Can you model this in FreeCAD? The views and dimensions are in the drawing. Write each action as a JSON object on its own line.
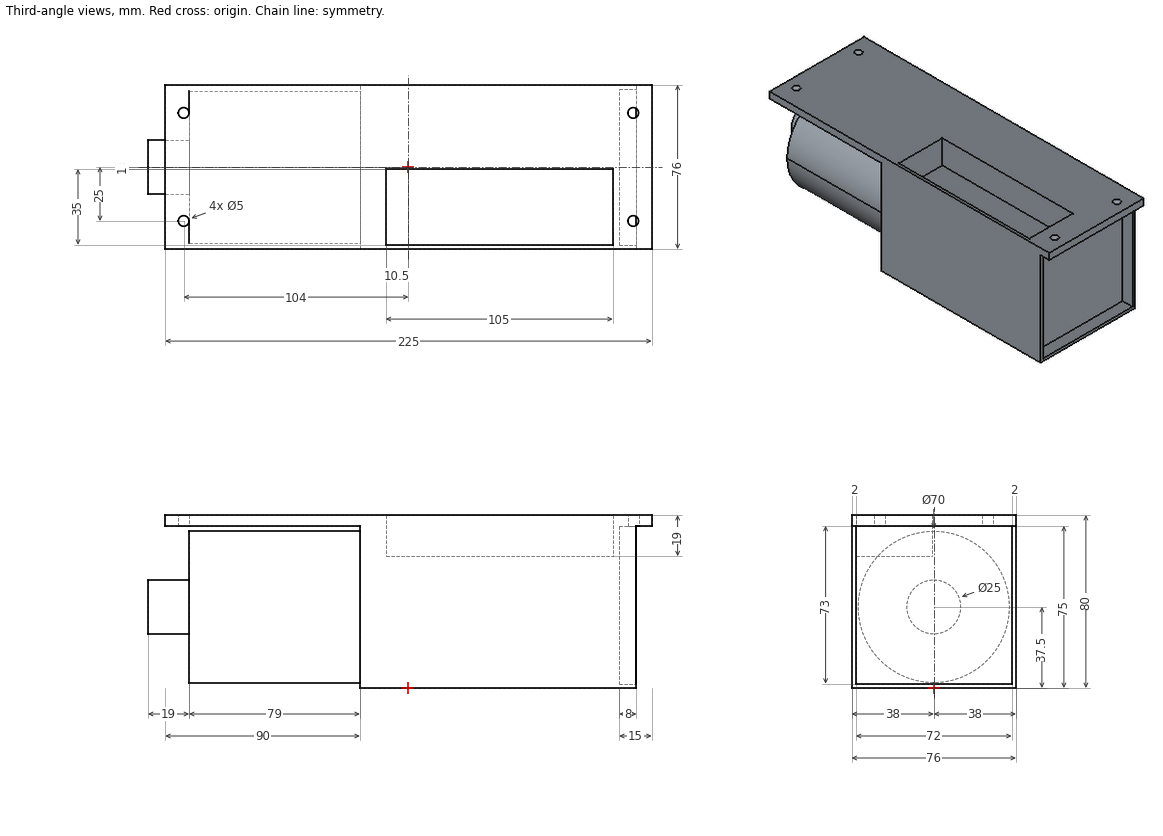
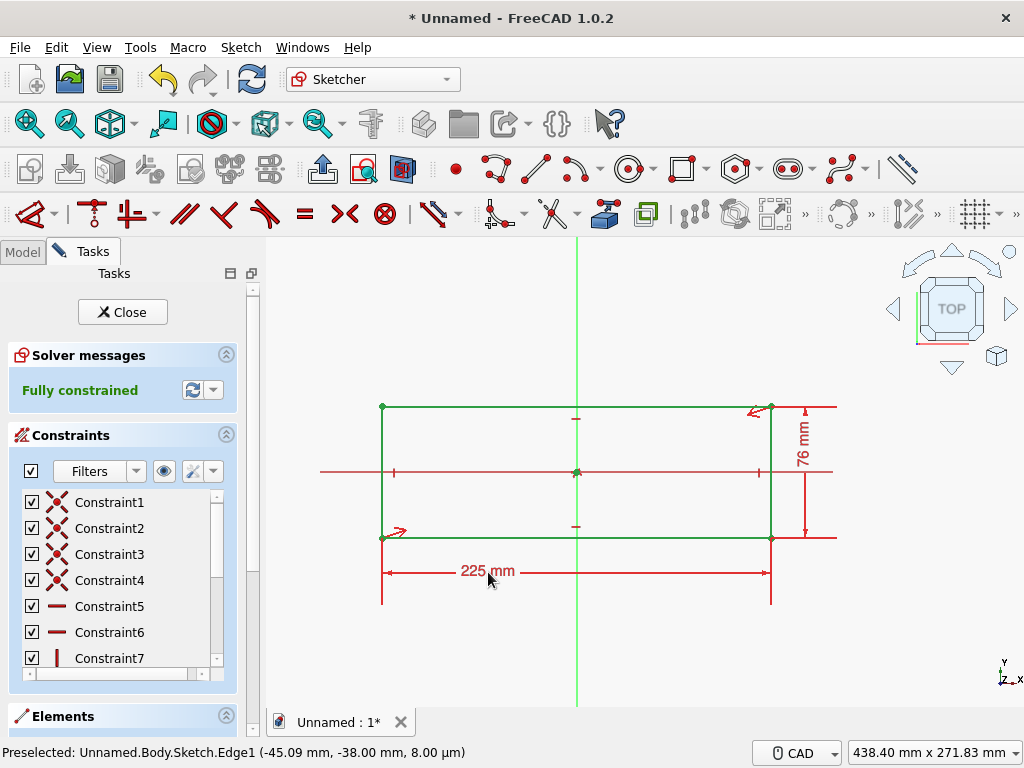
{"action": "left_click", "coordinate": [123, 312]}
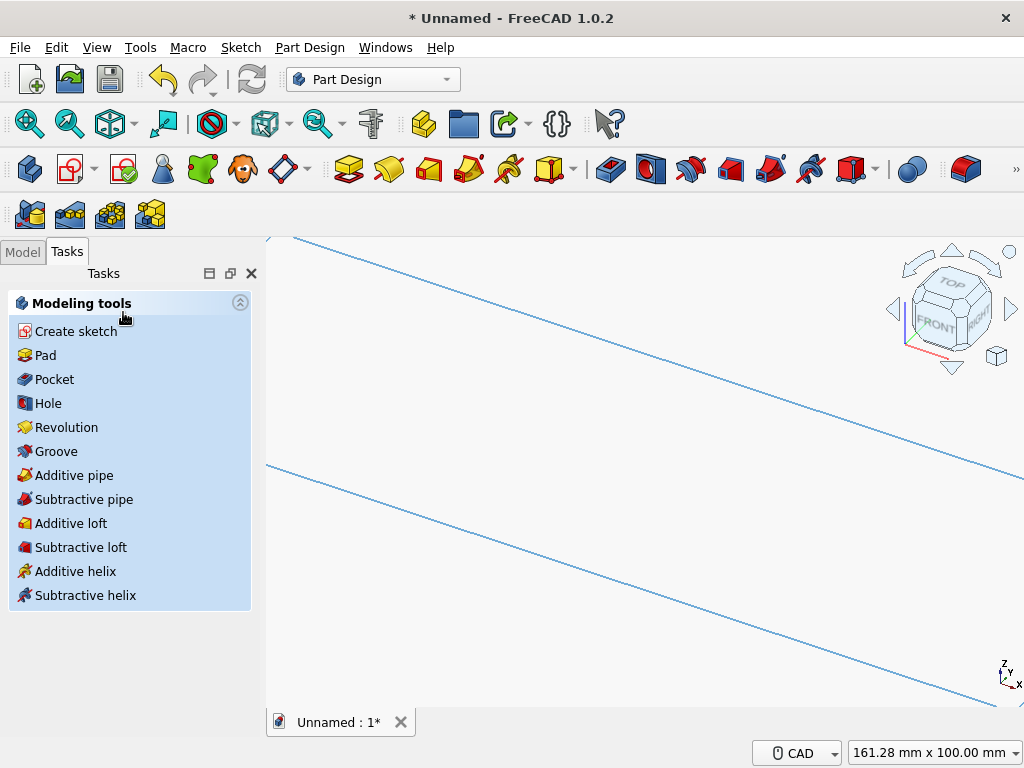
{"action": "left_click", "coordinate": [350, 170]}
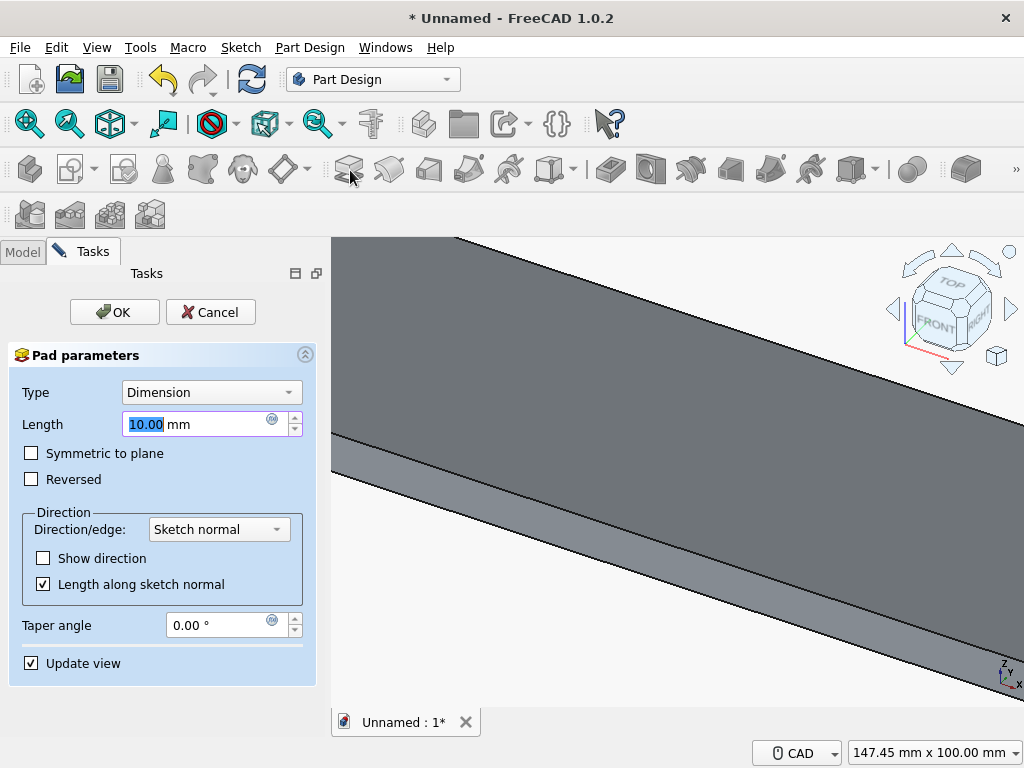
{"action": "type", "text": "80"}
{"action": "key", "text": "Tab"}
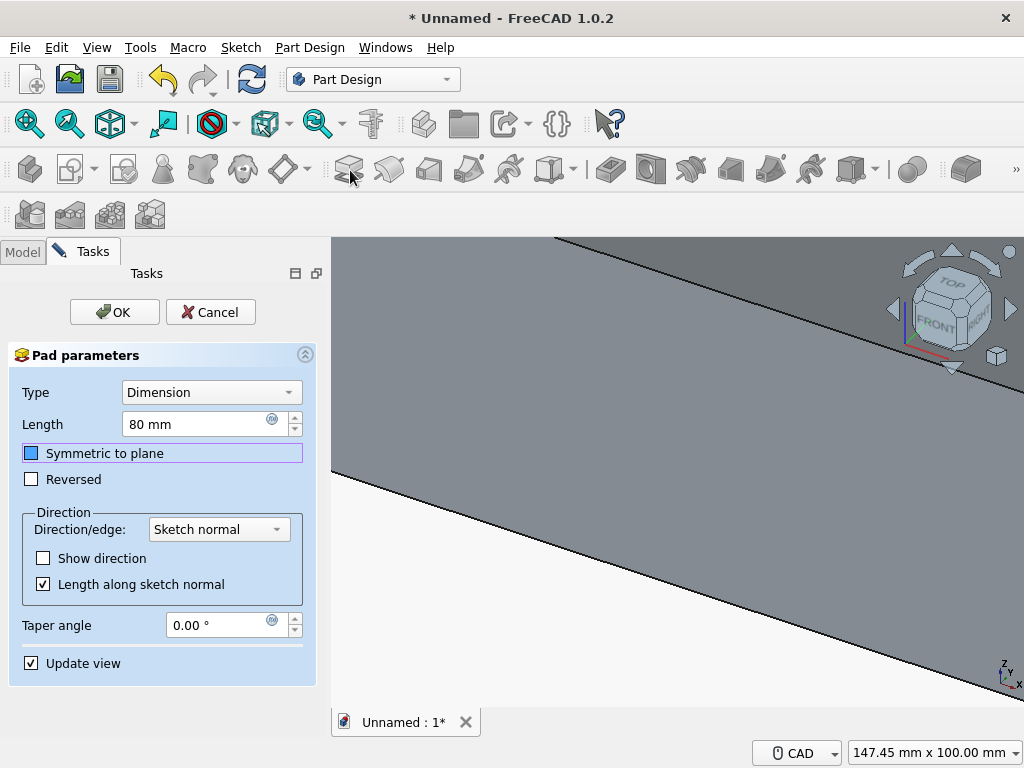
{"action": "left_click", "coordinate": [115, 312]}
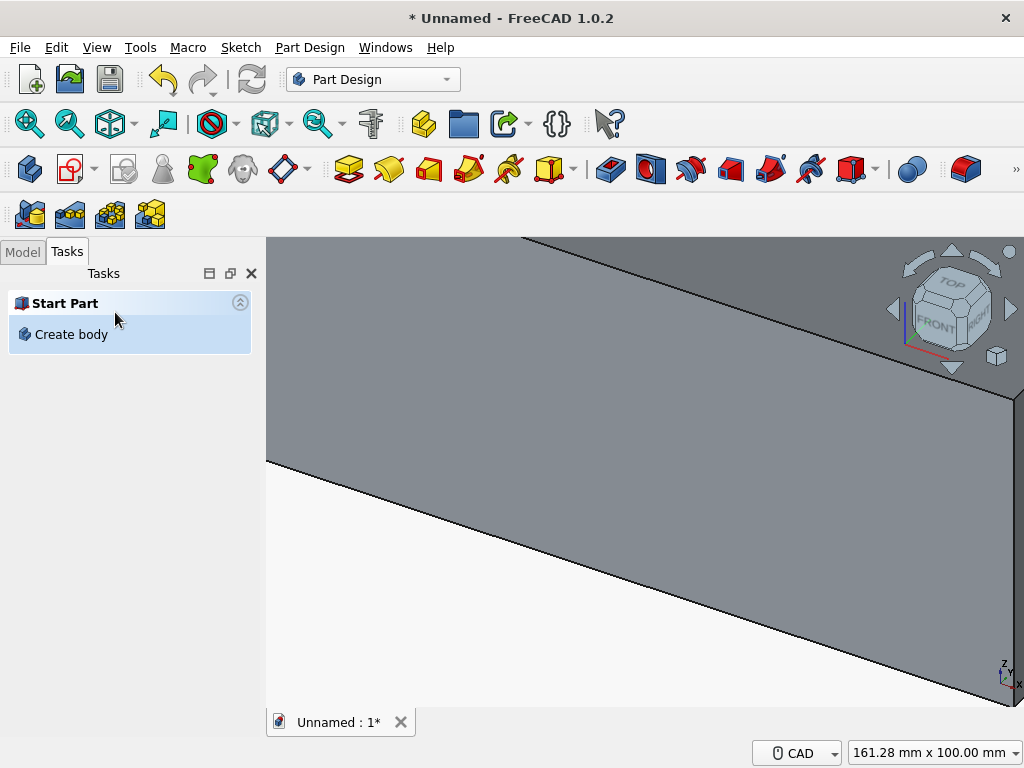
{"action": "key", "text": "v f"}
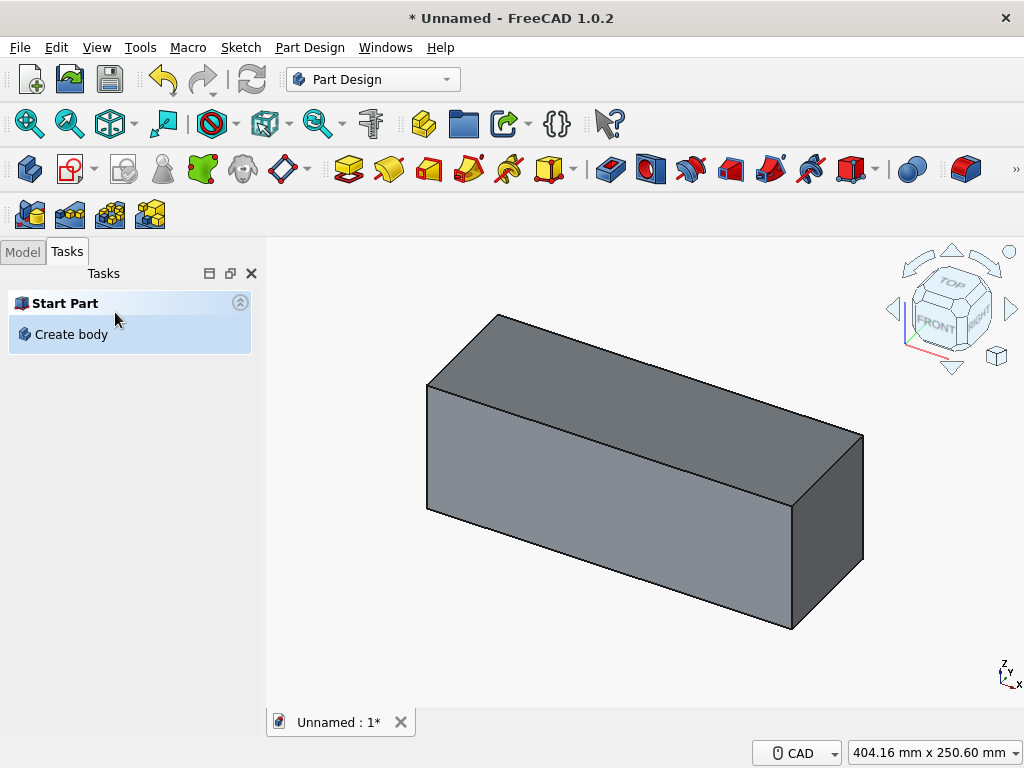
{"action": "key", "text": "6"}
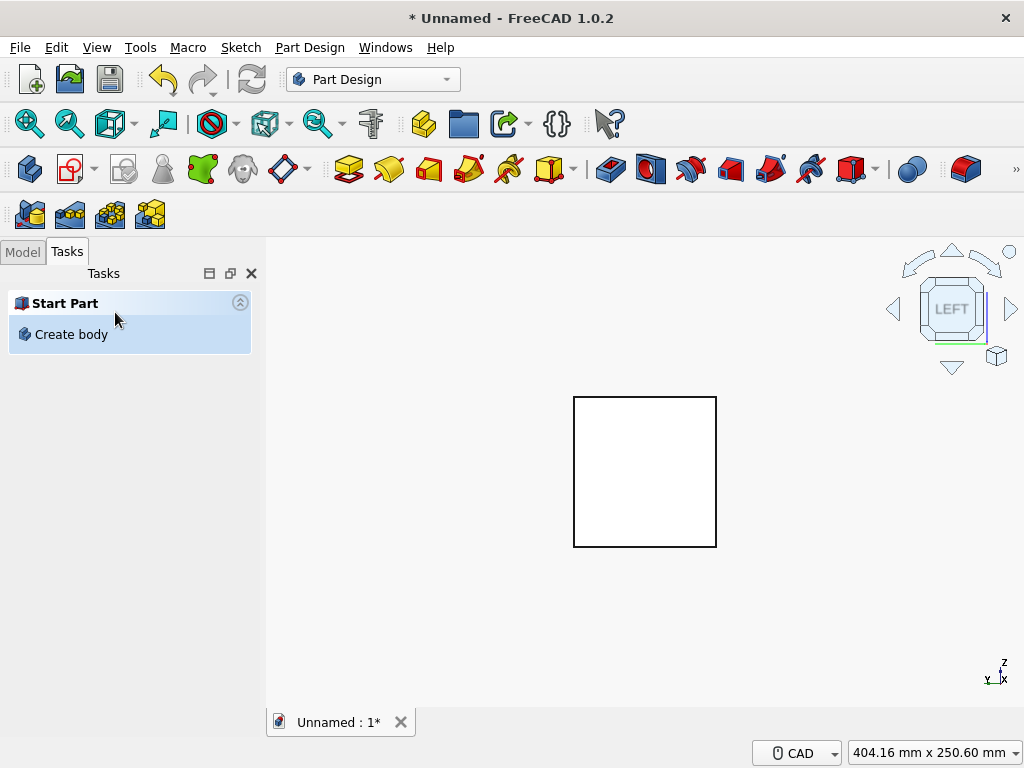
{"action": "left_click", "coordinate": [30, 124]}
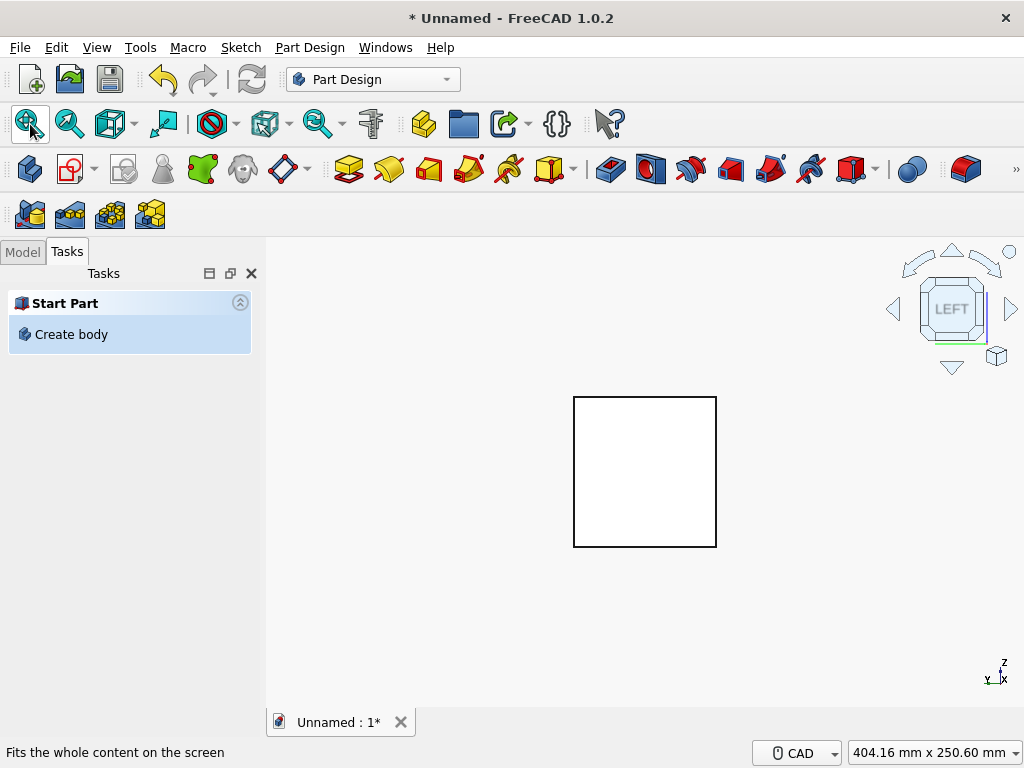
{"action": "left_click", "coordinate": [645, 471]}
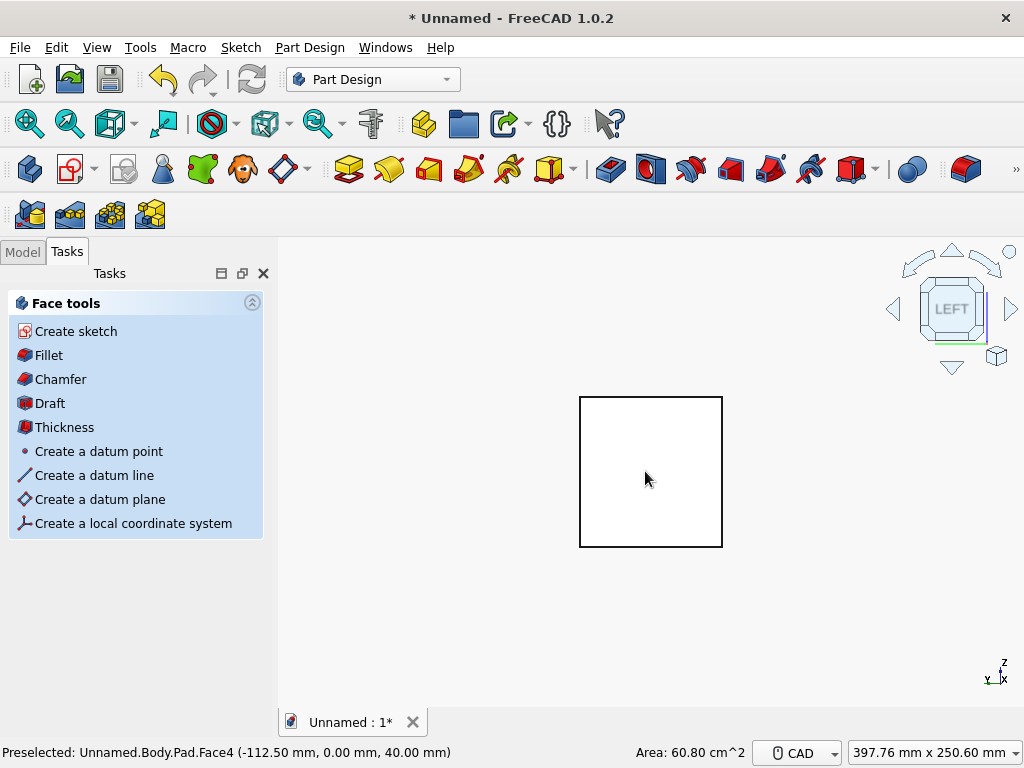
{"action": "left_click", "coordinate": [70, 170]}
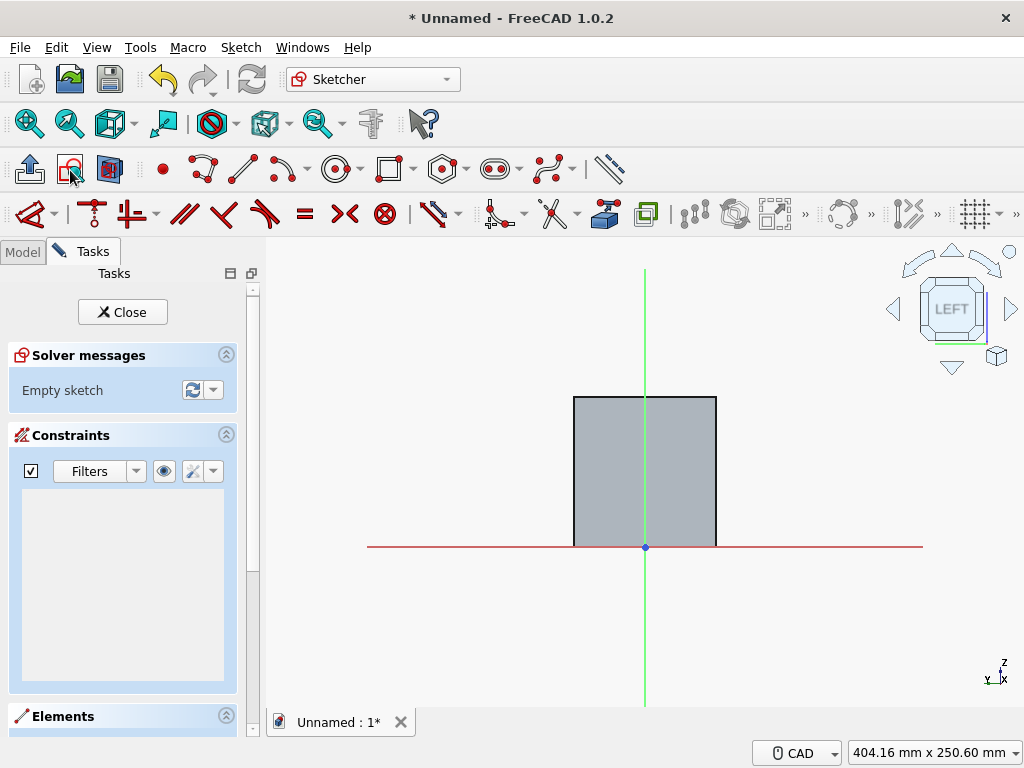
{"action": "scroll", "coordinate": [701, 481], "scroll_direction": "up", "scroll_amount": 4}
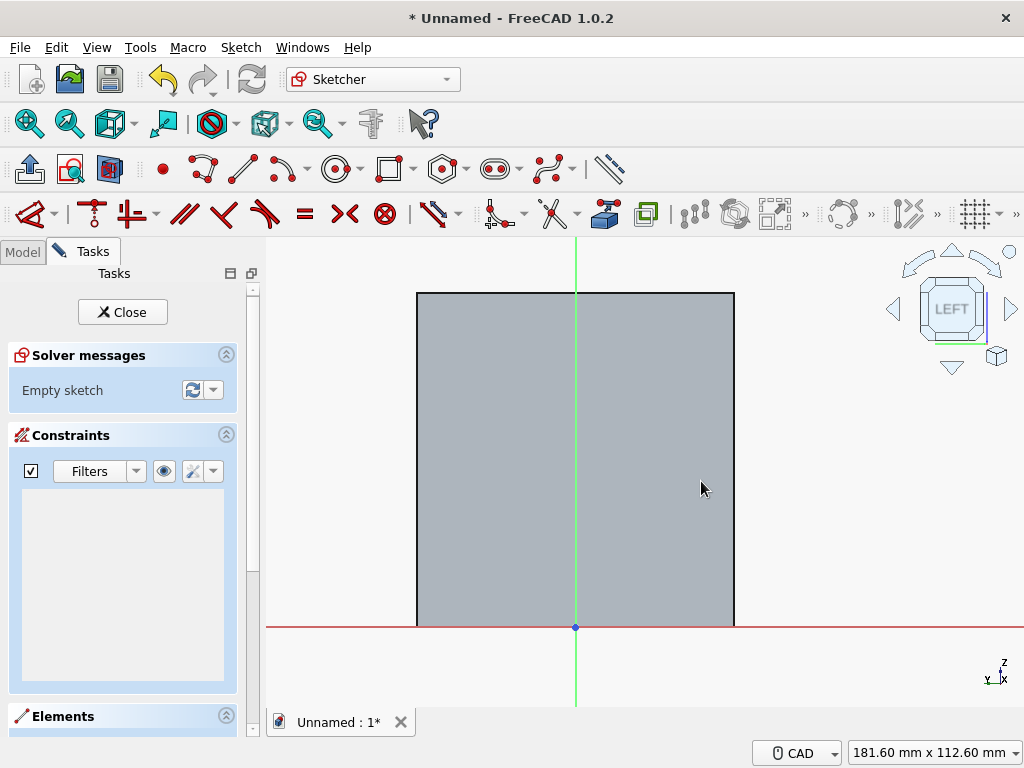
{"action": "key", "text": "g r"}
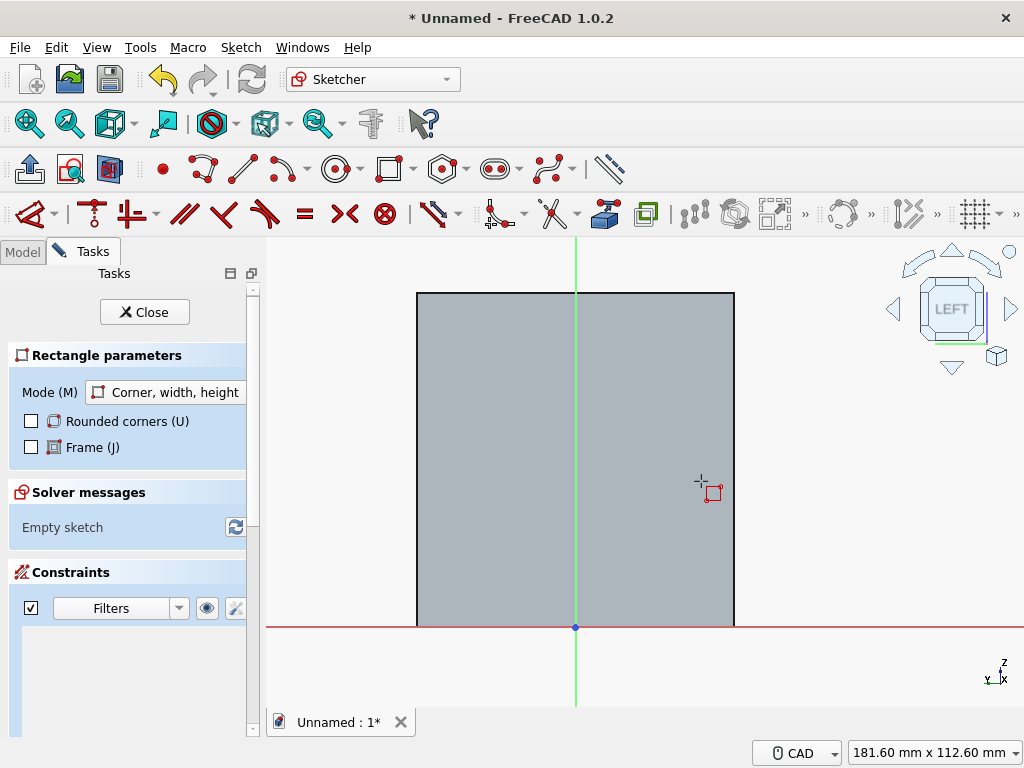
{"action": "left_click", "coordinate": [417, 314]}
{"action": "left_click", "coordinate": [734, 627]}
{"action": "key", "text": "Escape"}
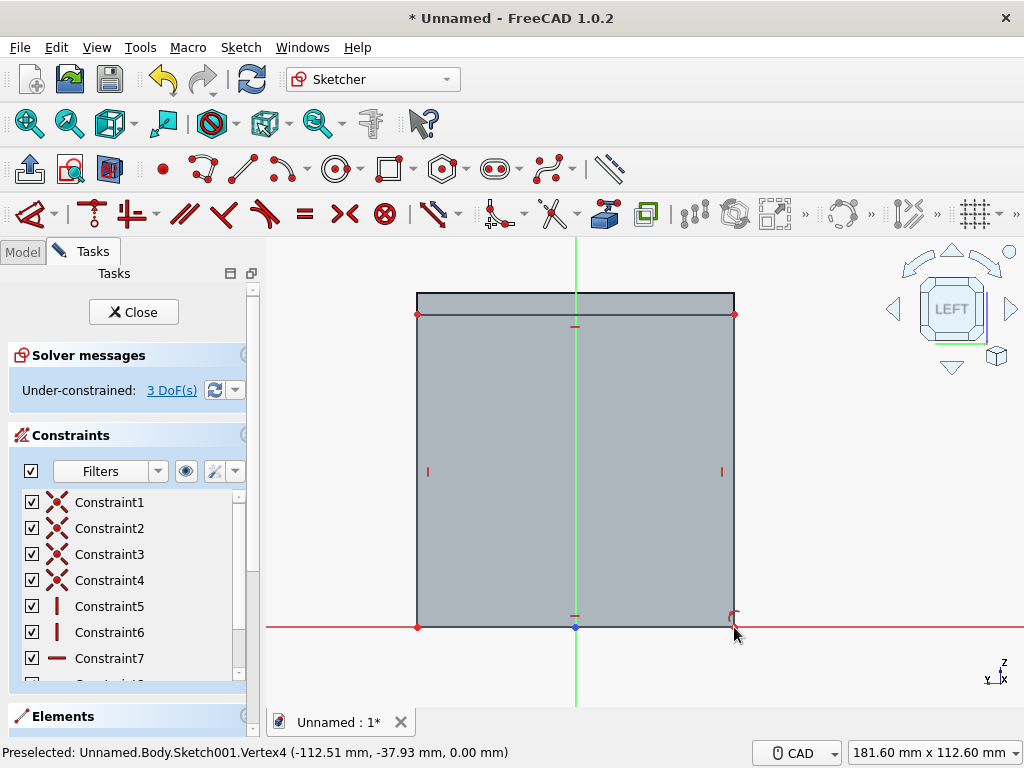
{"action": "left_click", "coordinate": [30, 214]}